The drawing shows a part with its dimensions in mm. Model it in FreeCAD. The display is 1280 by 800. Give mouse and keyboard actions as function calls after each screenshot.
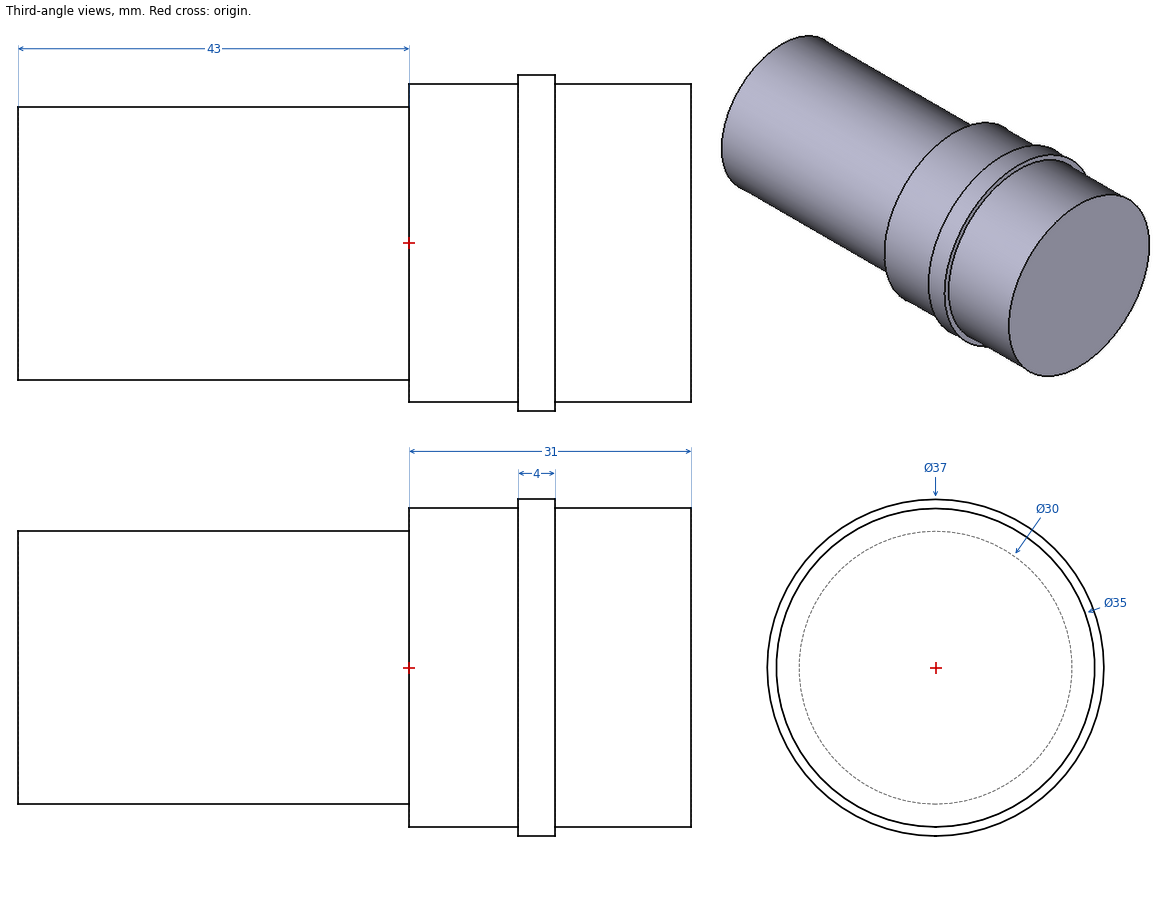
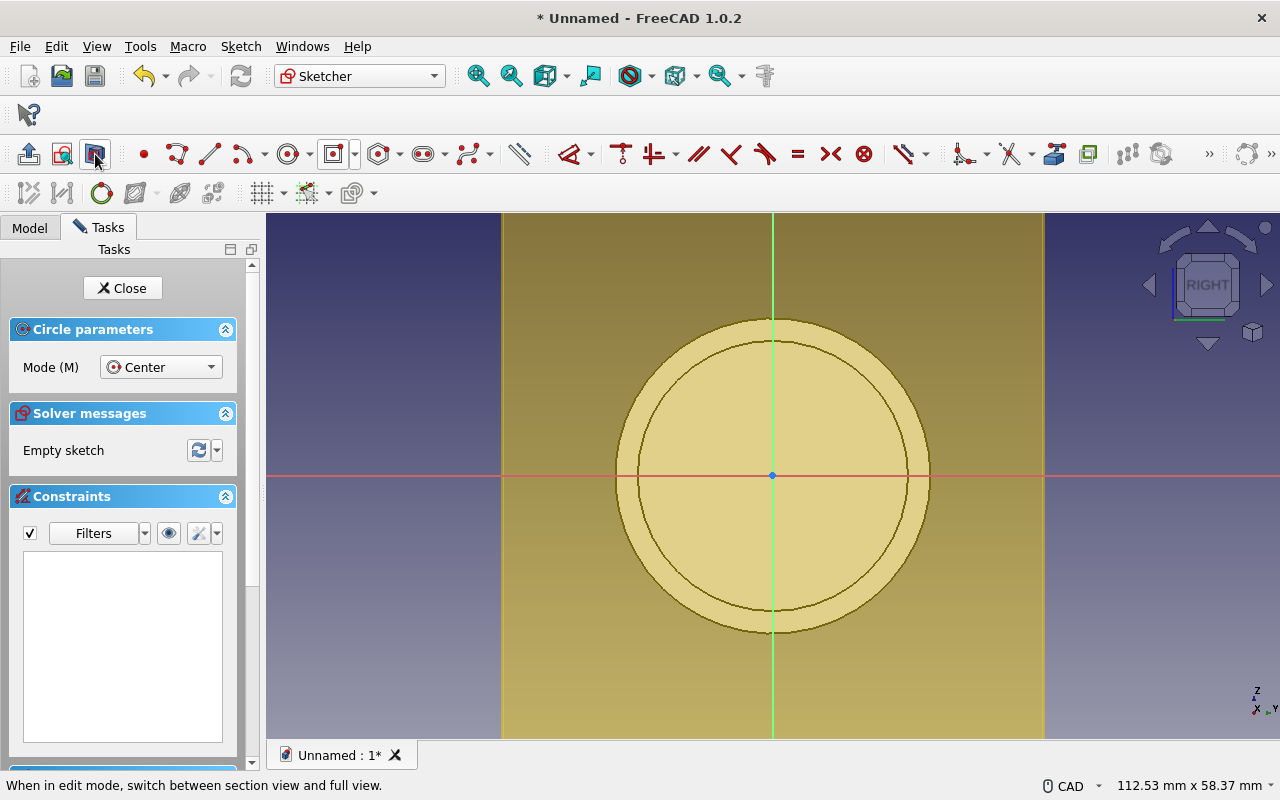
click(773, 476)
click(891, 358)
key(Escape)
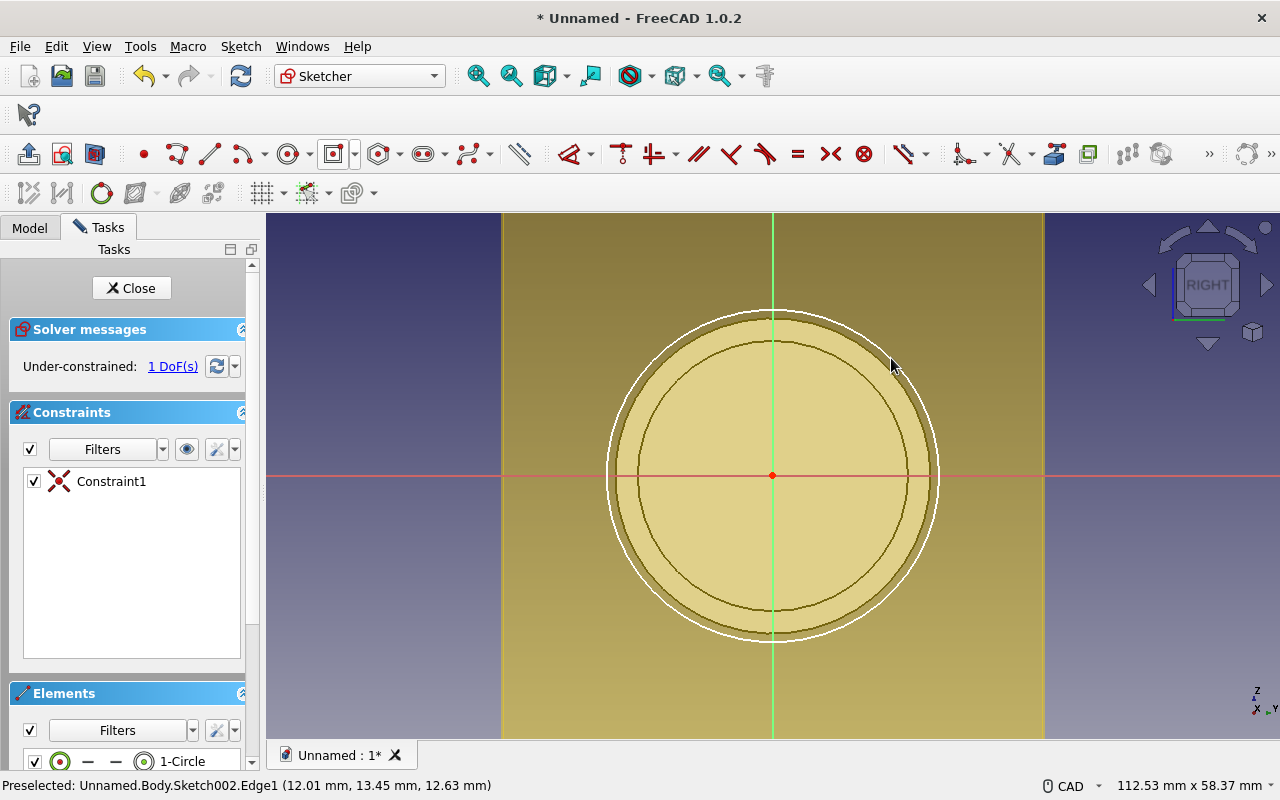
click(568, 154)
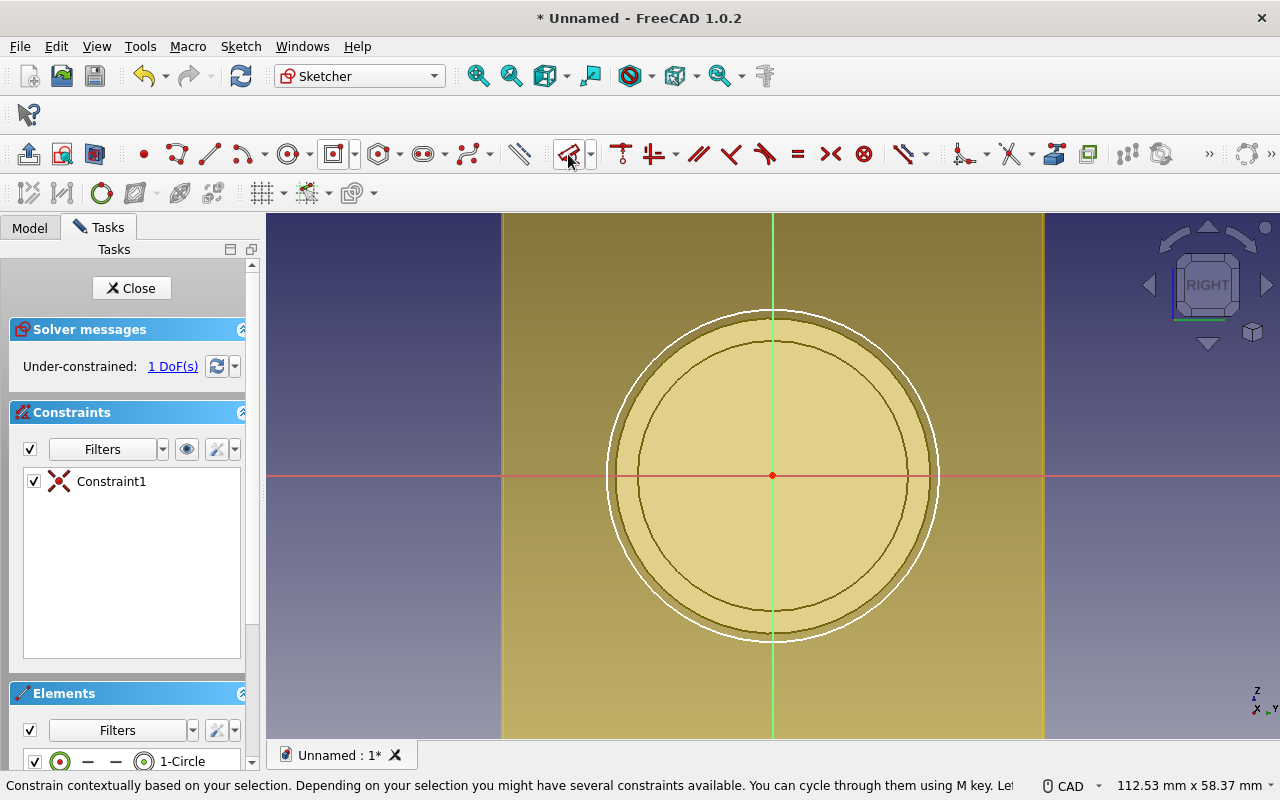
click(890, 358)
click(913, 335)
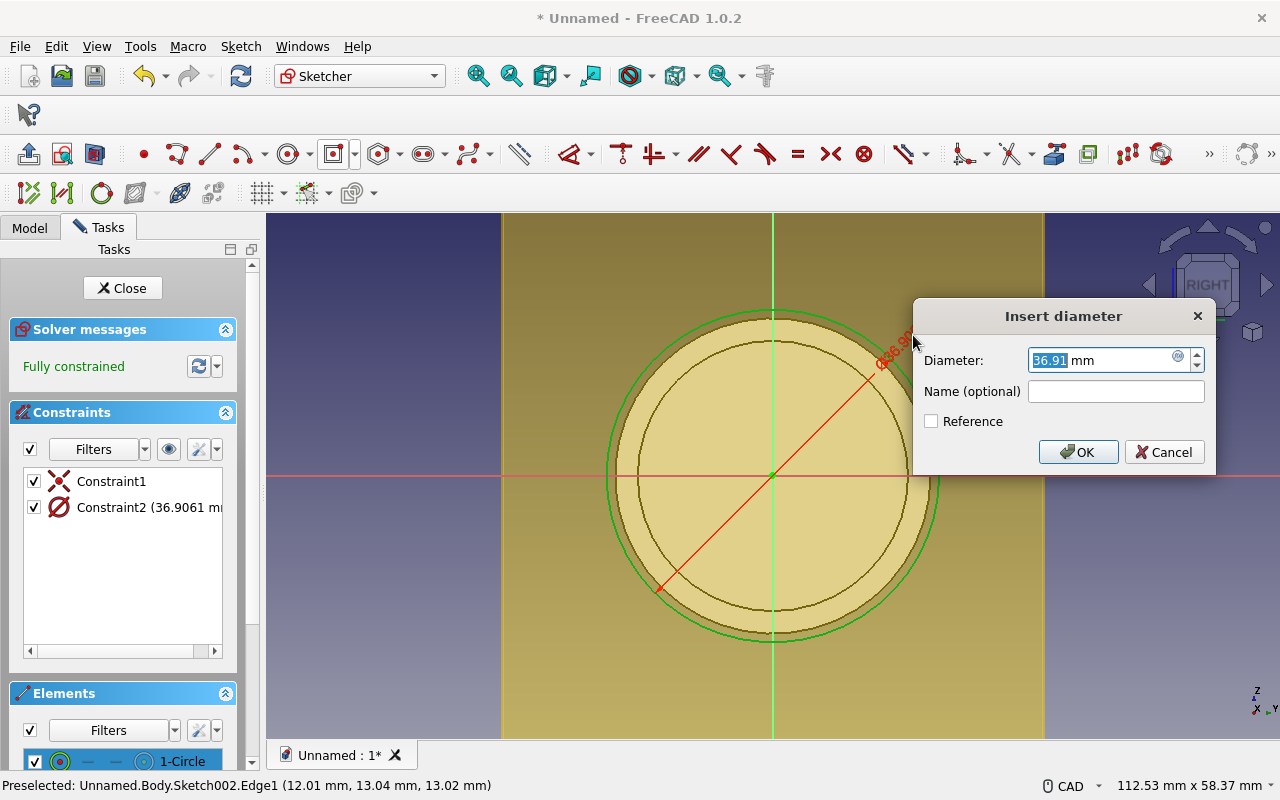
text(37)
key(Return)
key(Escape)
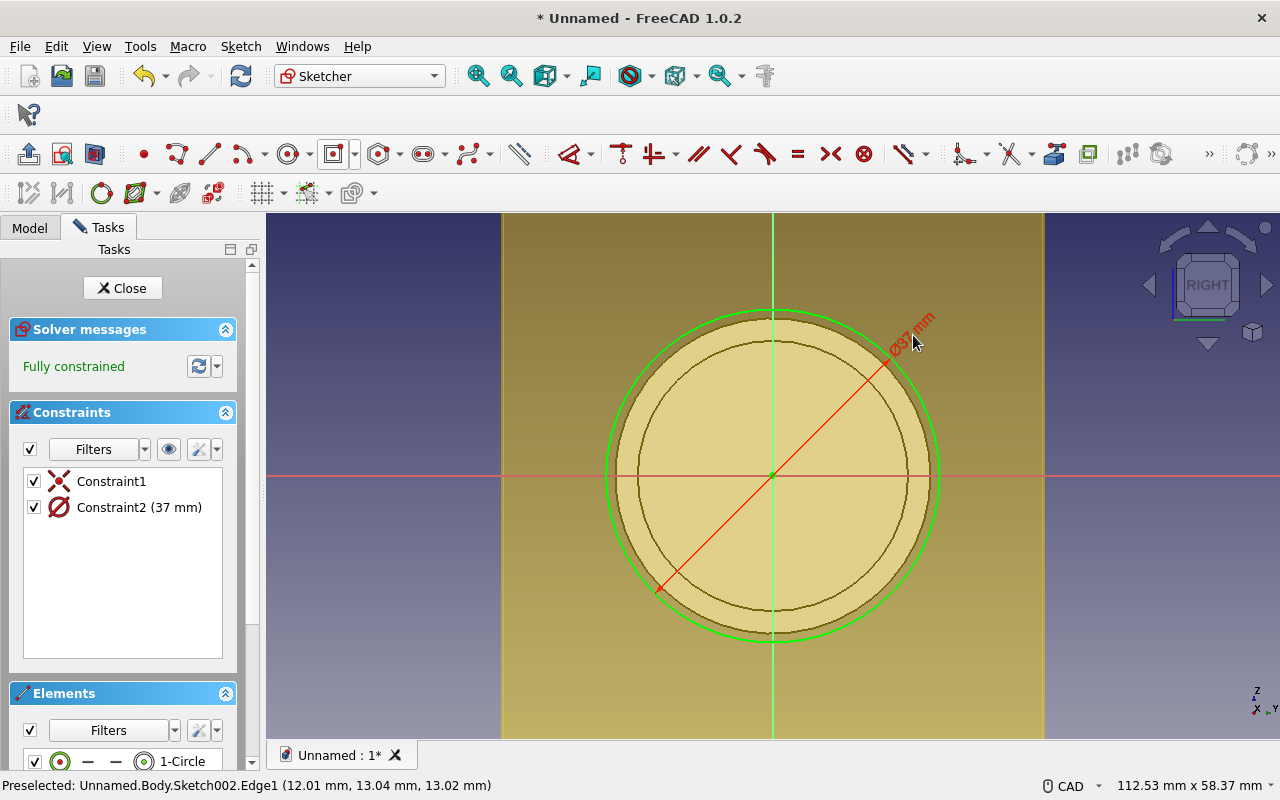
click(123, 288)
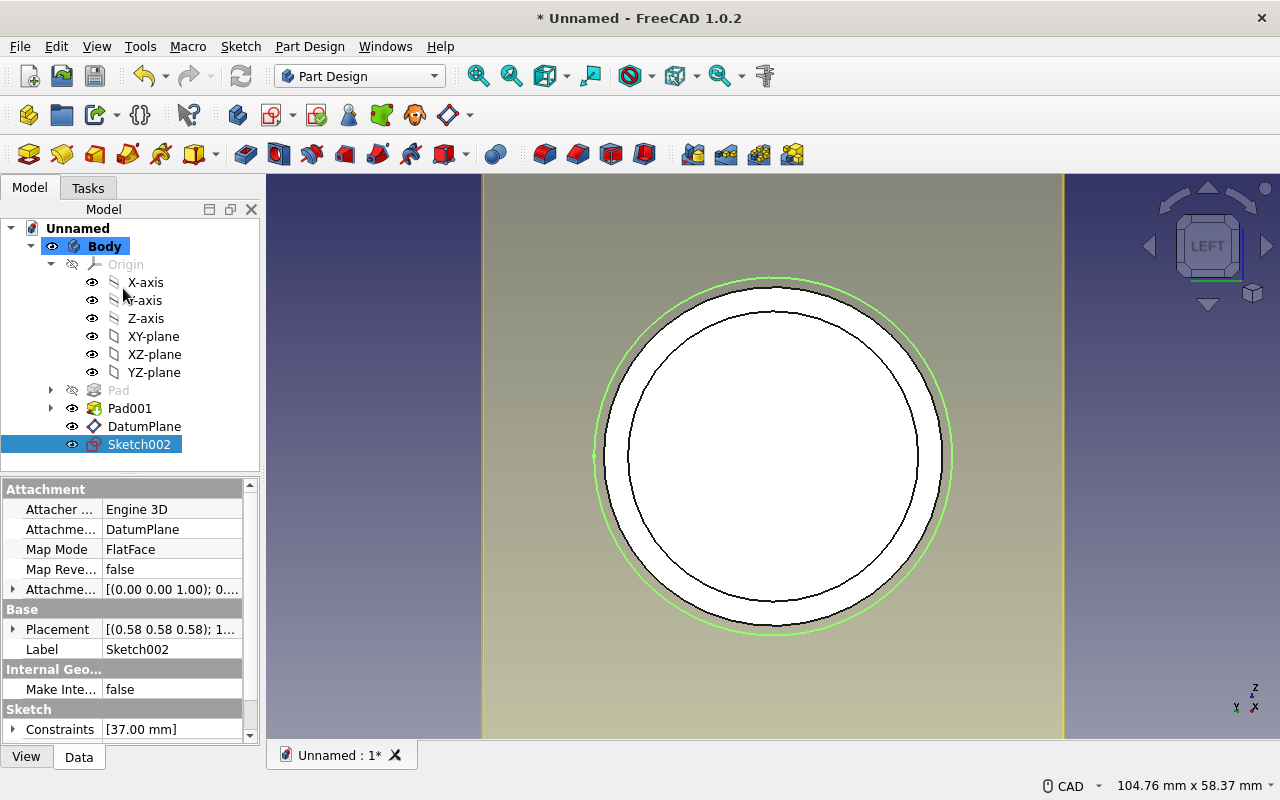
click(29, 154)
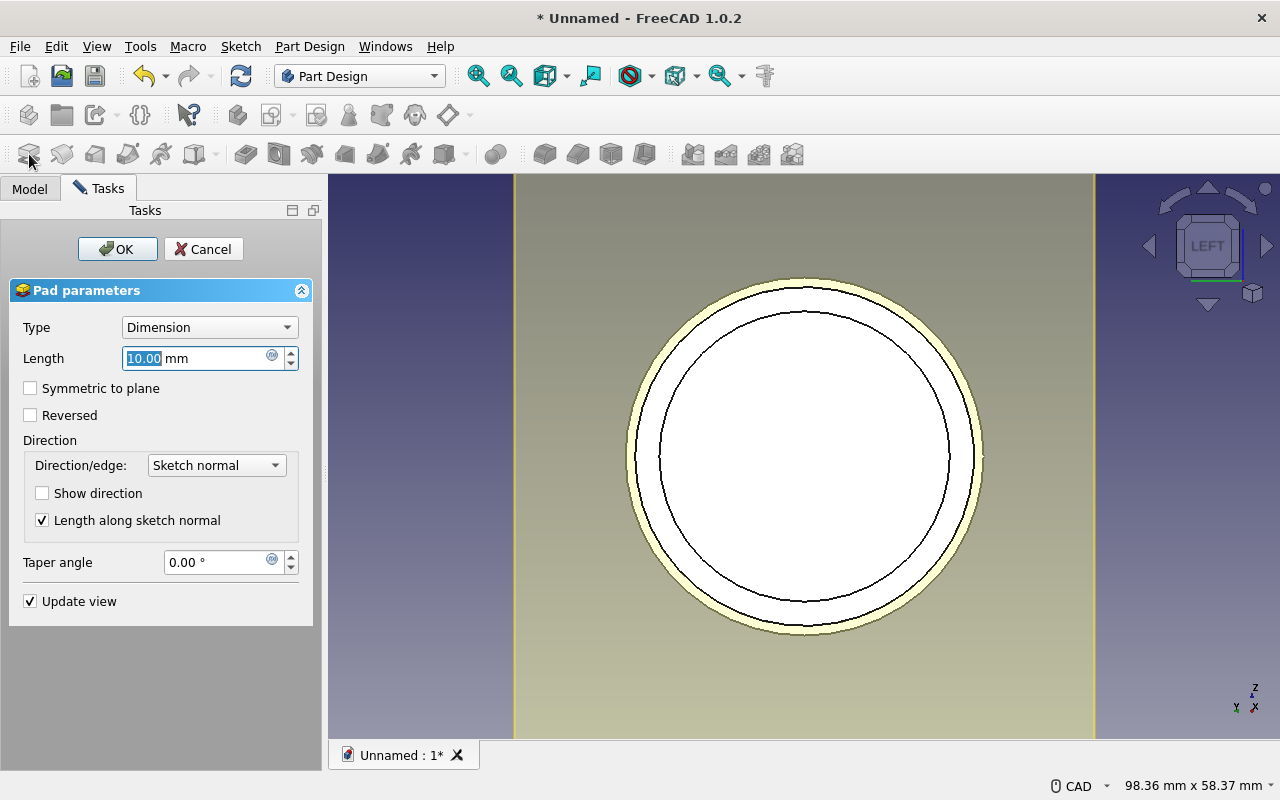
text(4)
key(Tab)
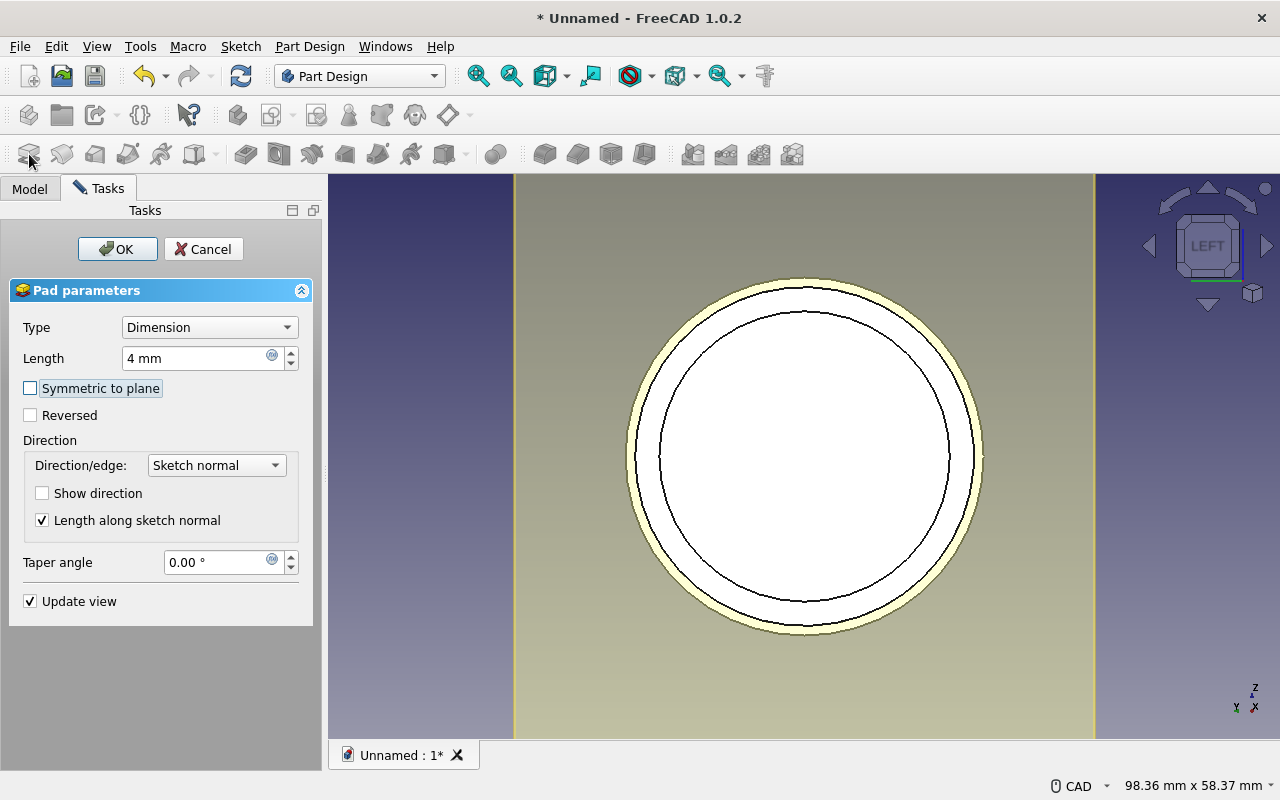
click(118, 249)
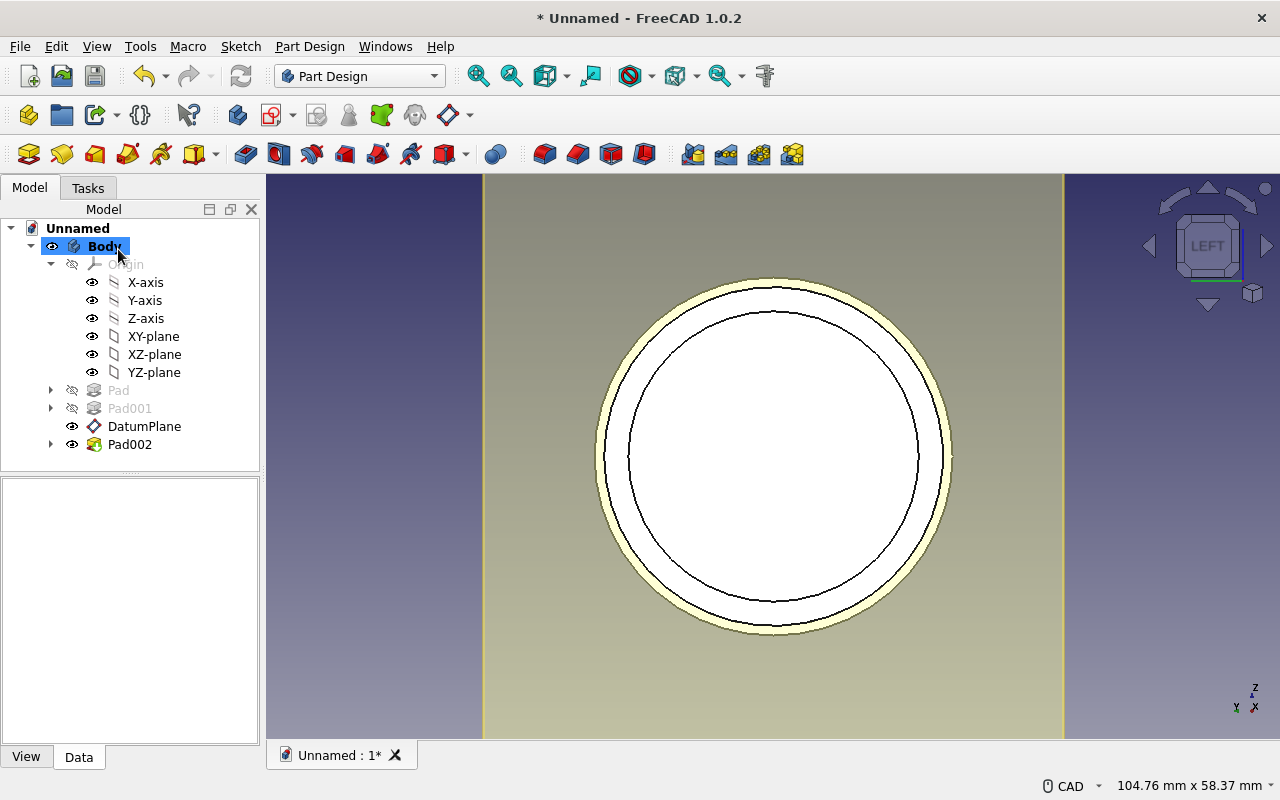
click(117, 426)
key(space)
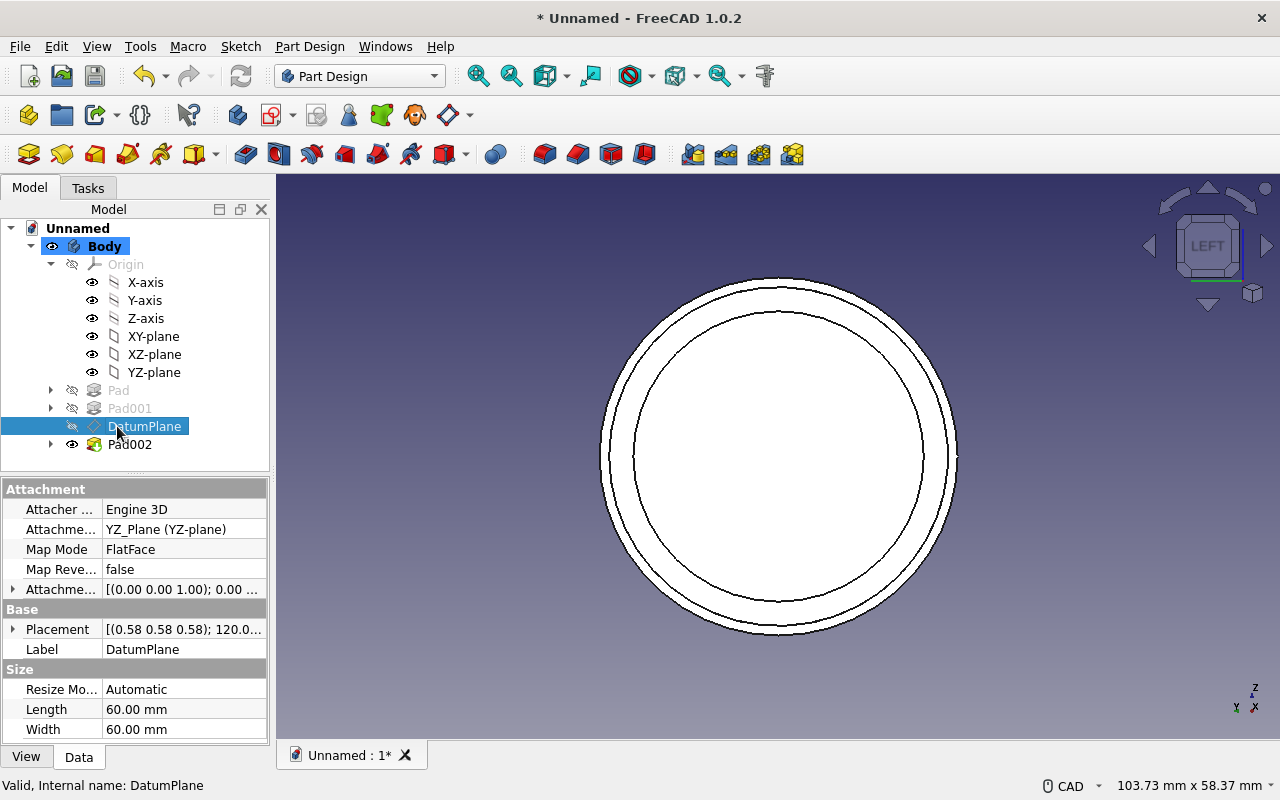
key(0)